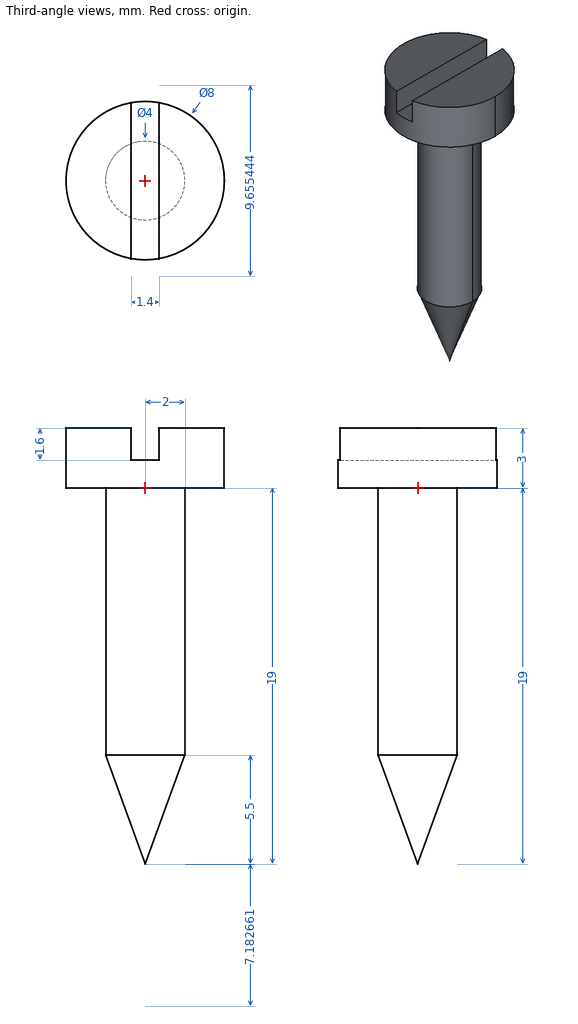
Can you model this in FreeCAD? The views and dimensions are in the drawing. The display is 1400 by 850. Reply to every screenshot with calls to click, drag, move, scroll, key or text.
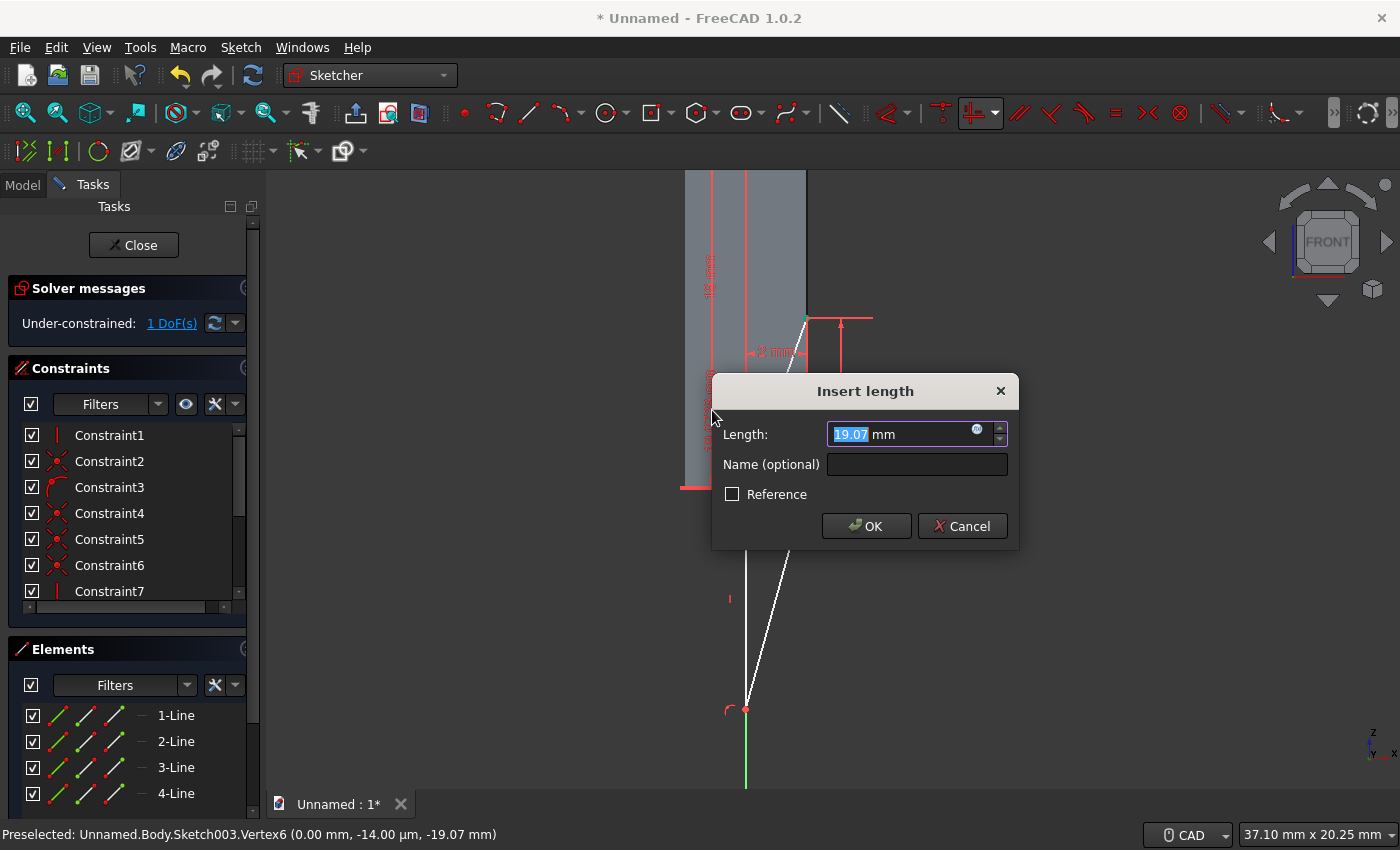
text(19)
key(Return)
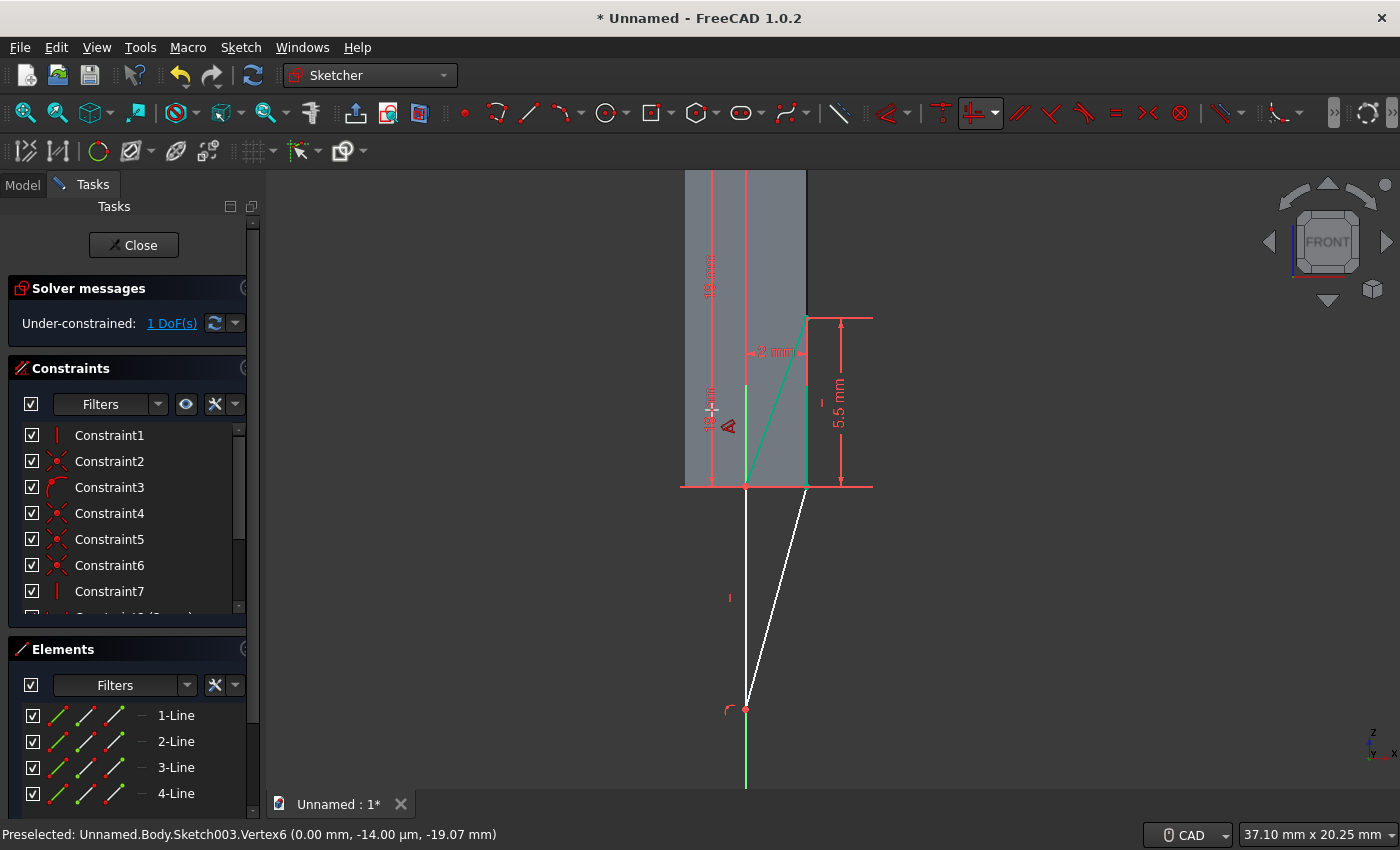
click(746, 642)
click(712, 598)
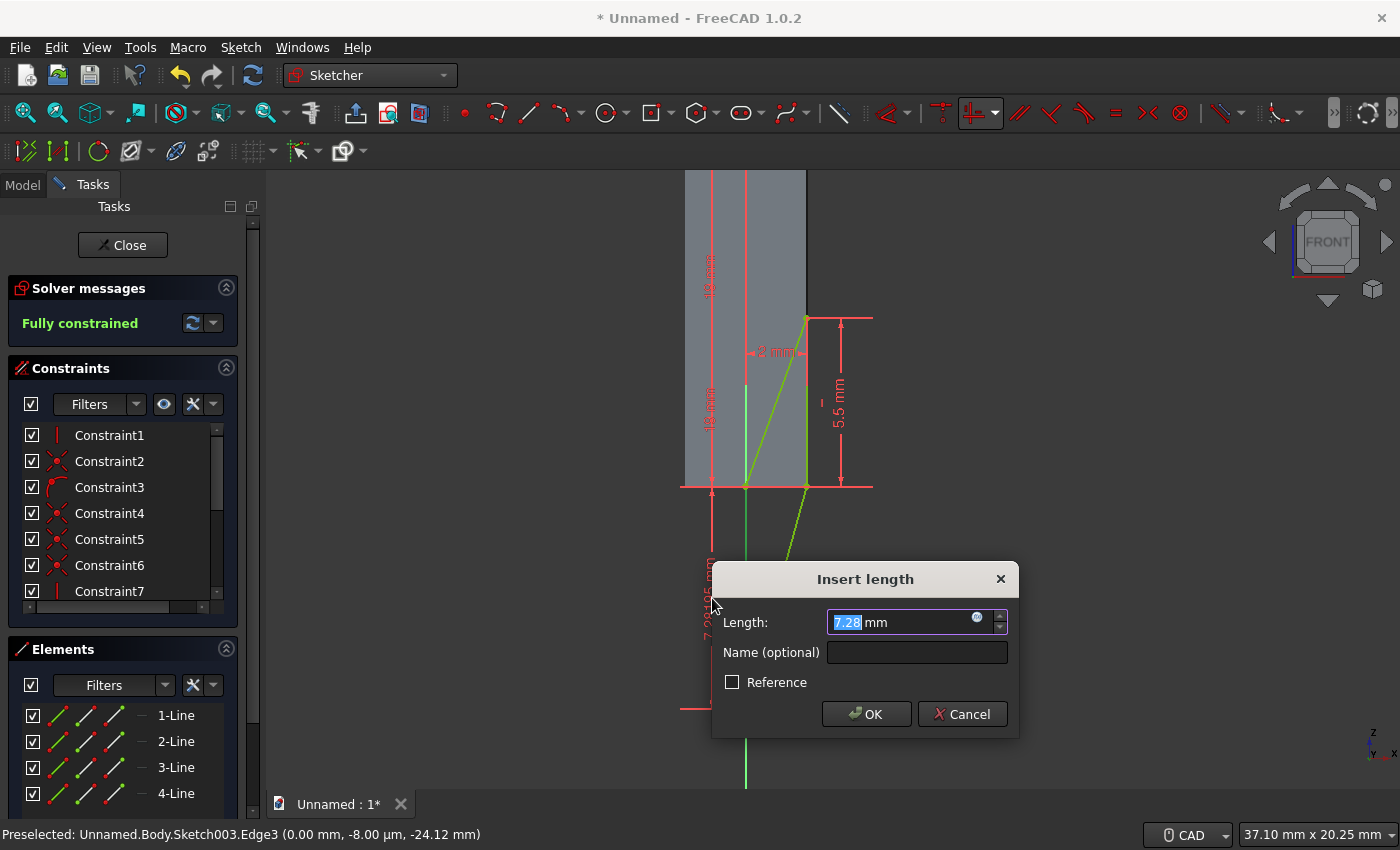
text(7.182661)
key(Return)
key(Escape)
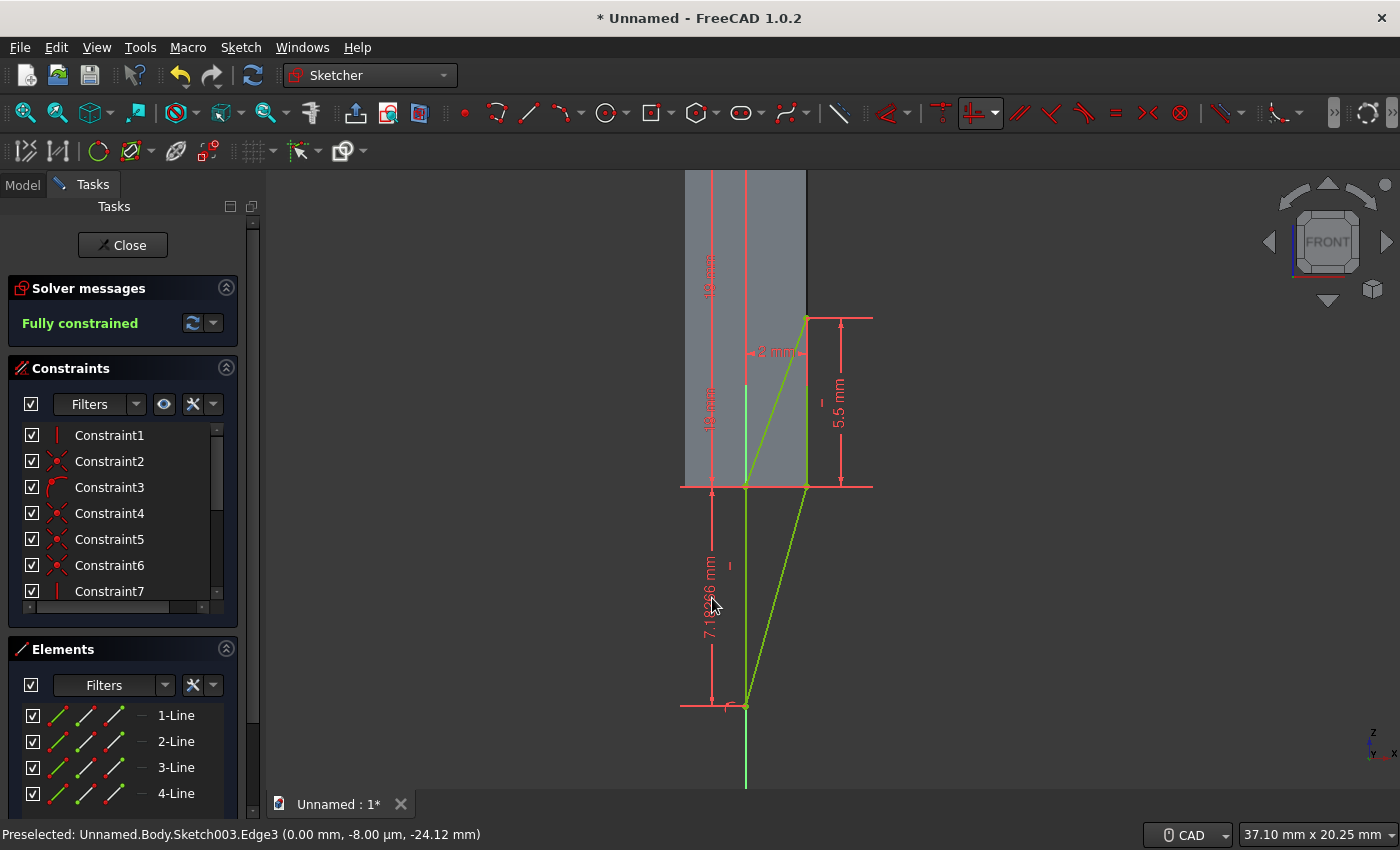
click(123, 245)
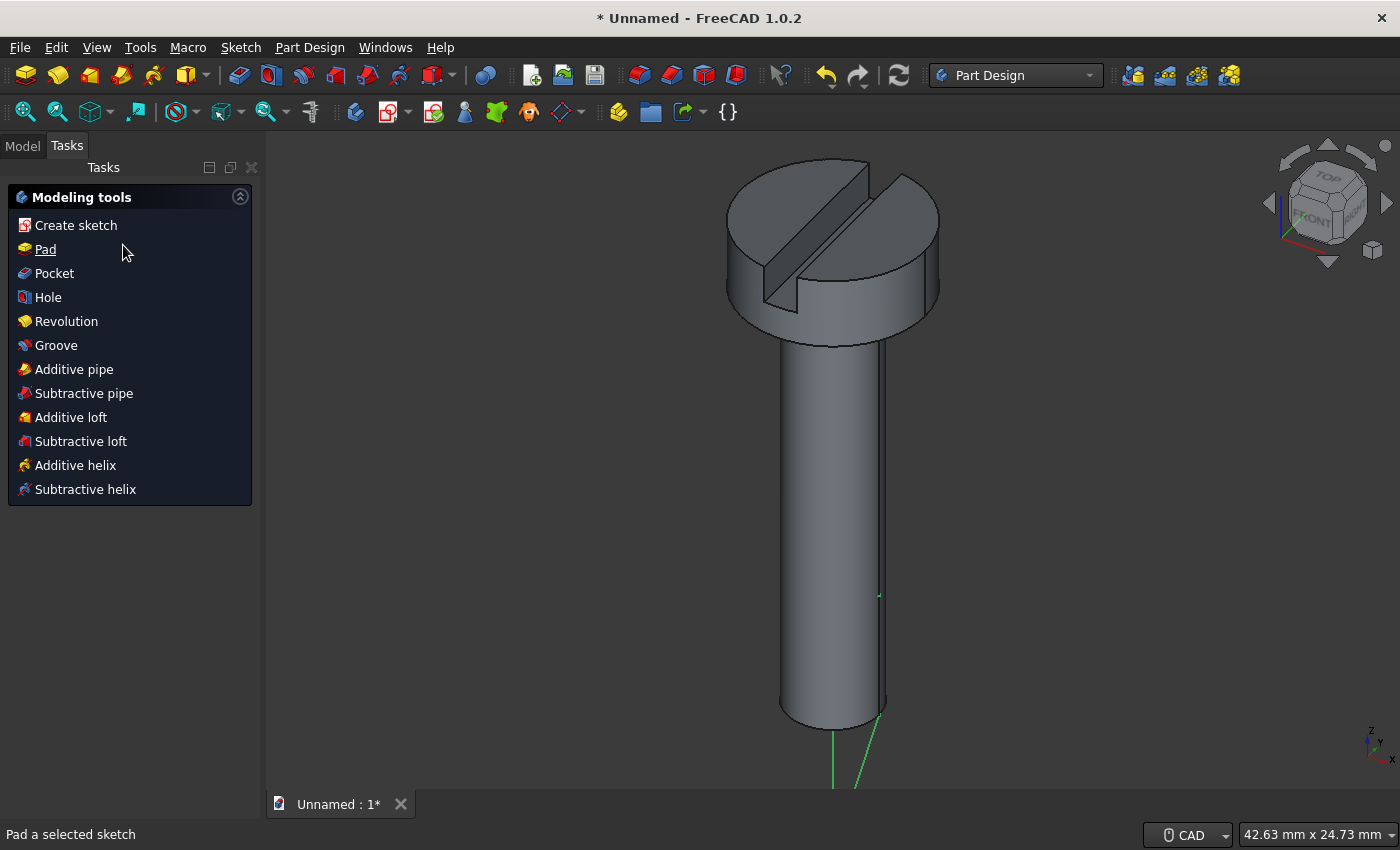
click(304, 76)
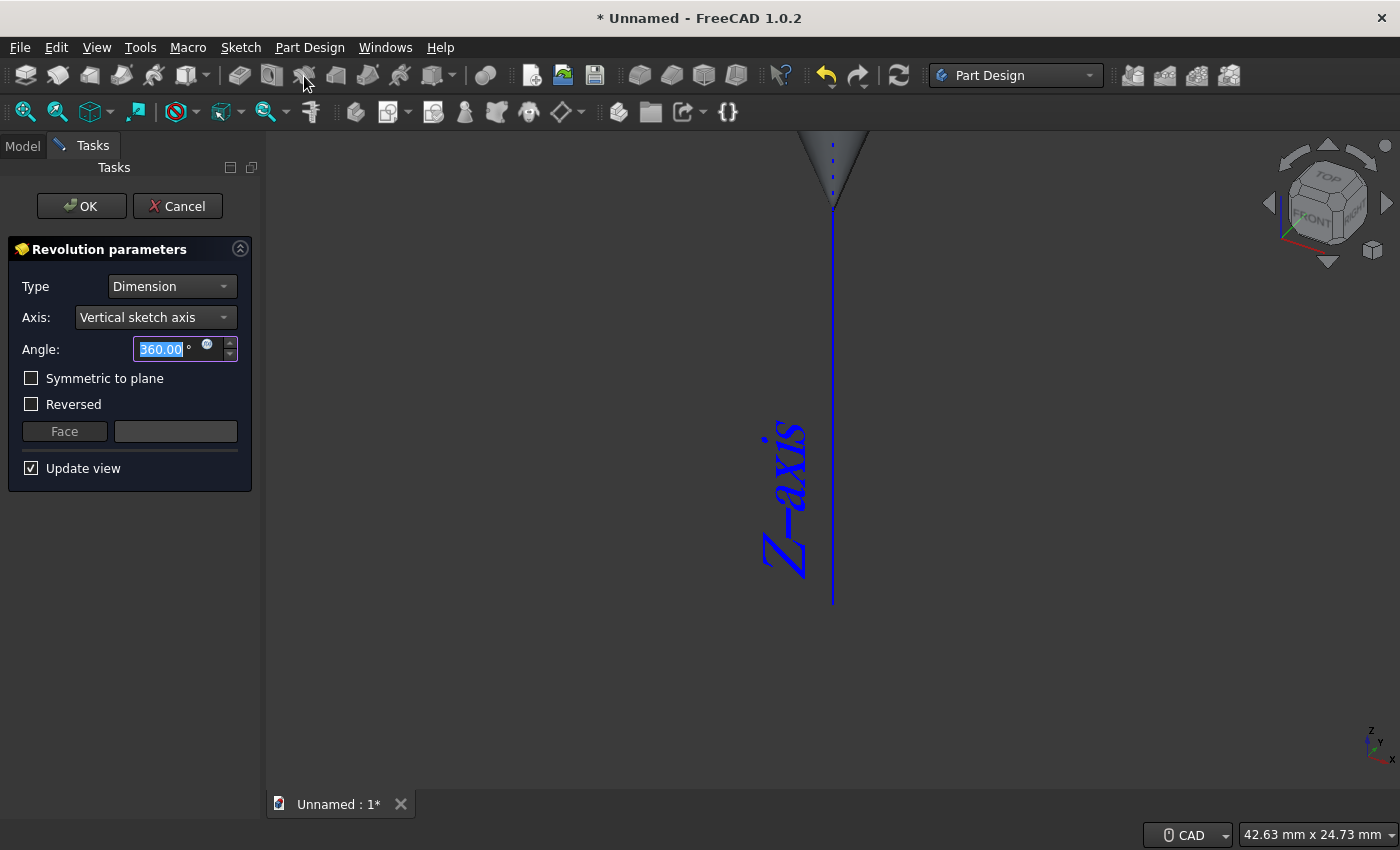
click(82, 206)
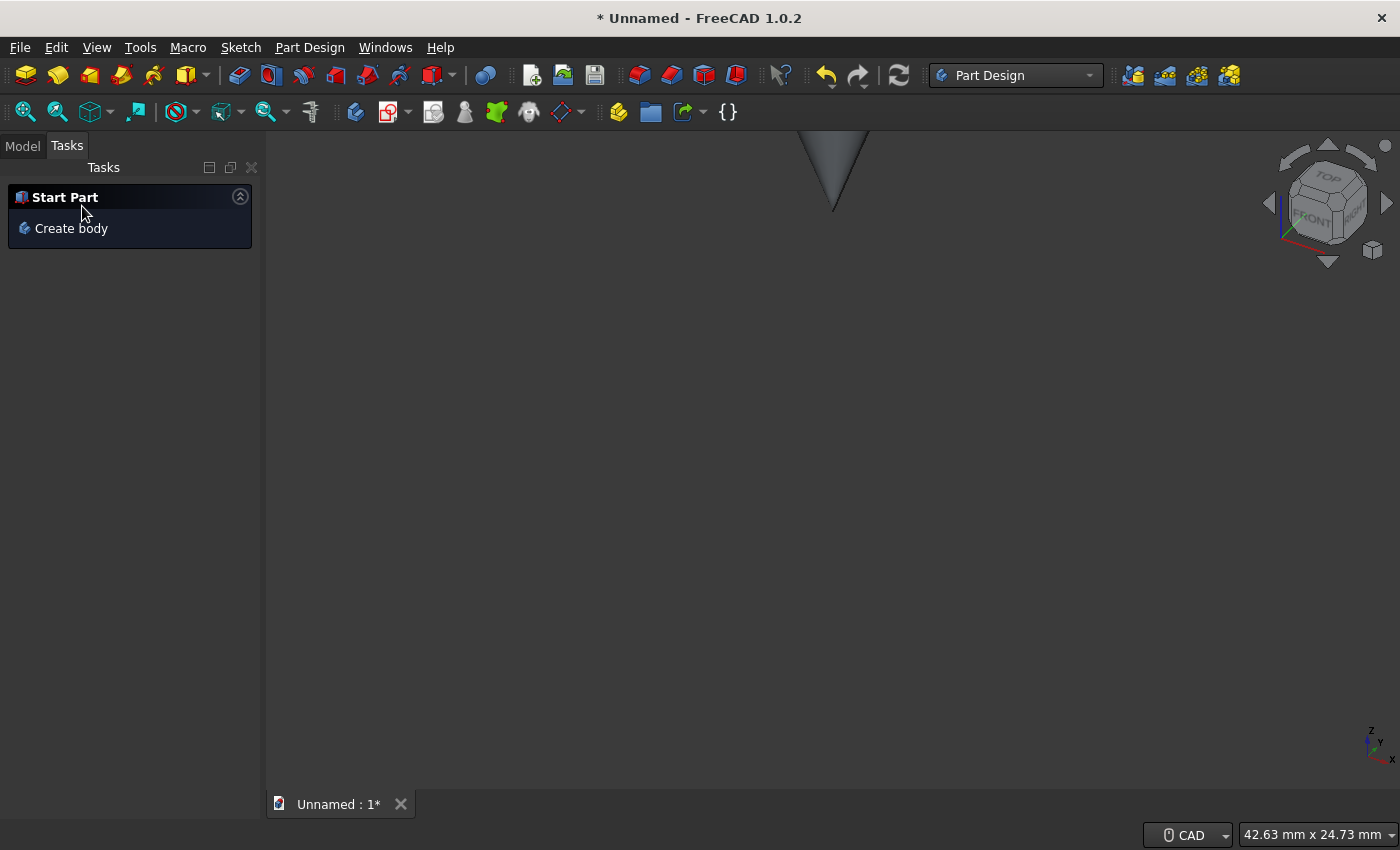
key(0)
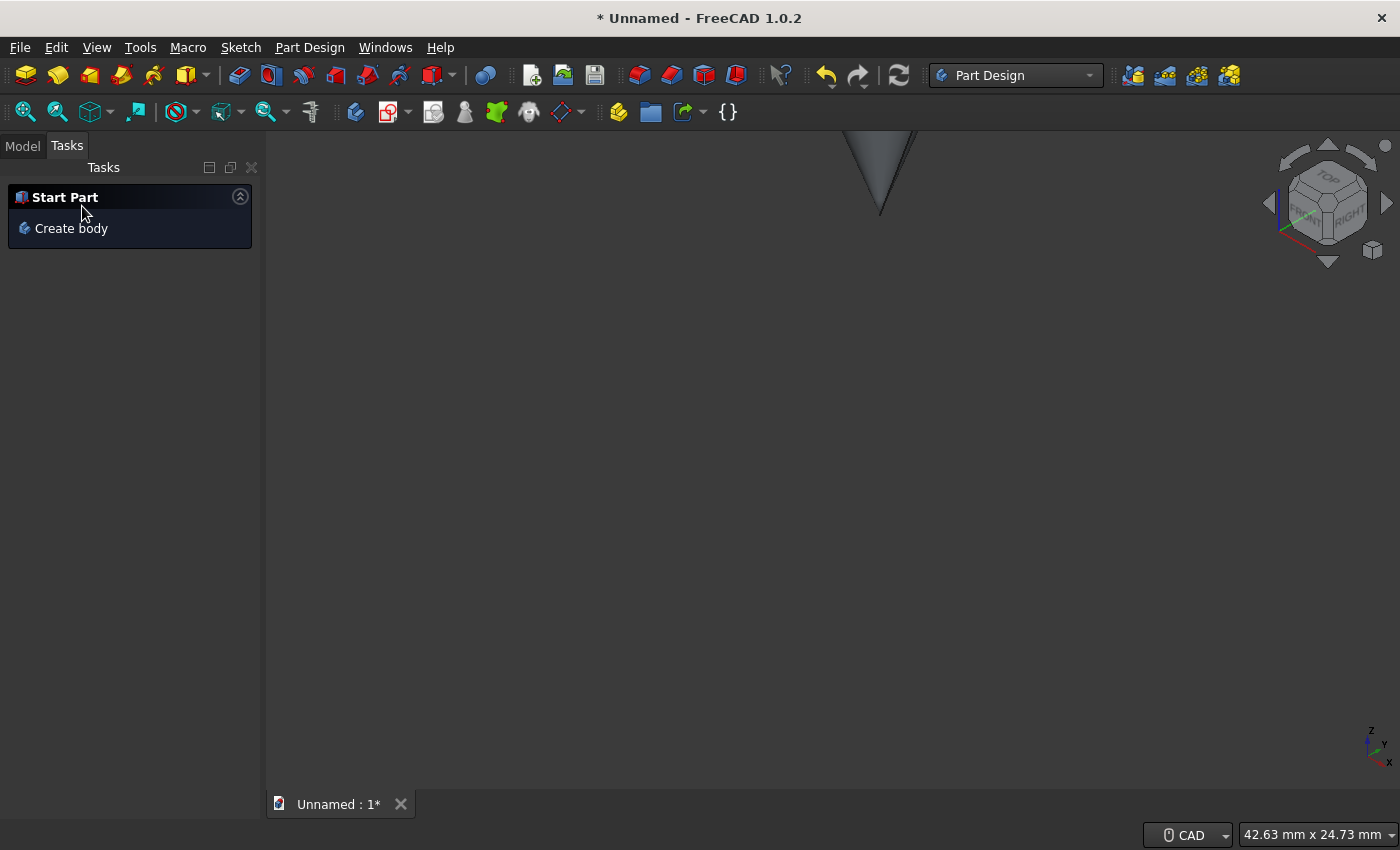
key(v)
key(f)